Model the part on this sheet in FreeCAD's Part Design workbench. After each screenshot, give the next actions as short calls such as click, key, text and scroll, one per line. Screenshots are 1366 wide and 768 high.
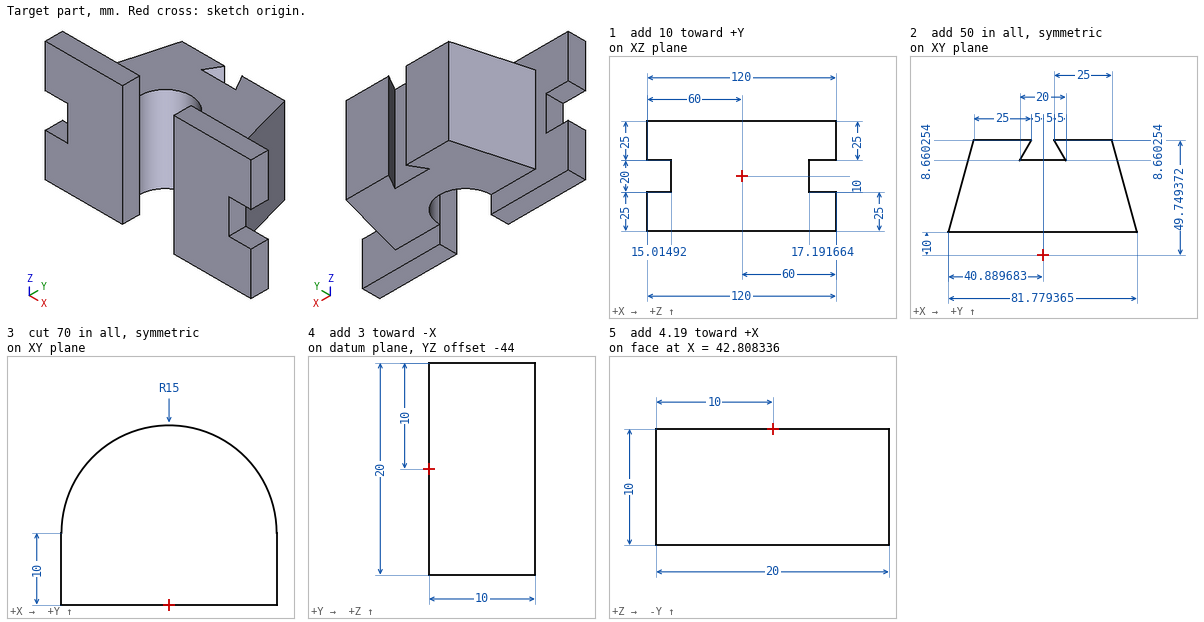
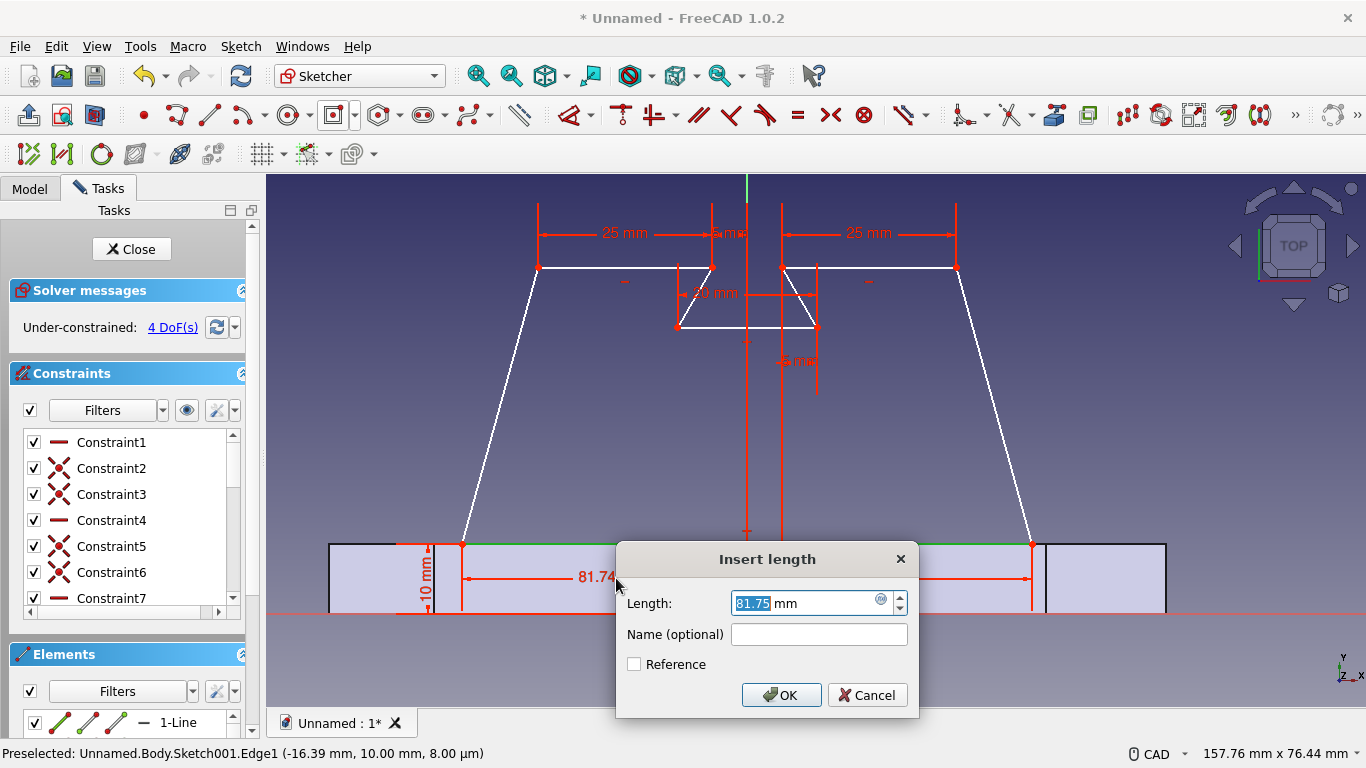
text(81.779365)
key(Return)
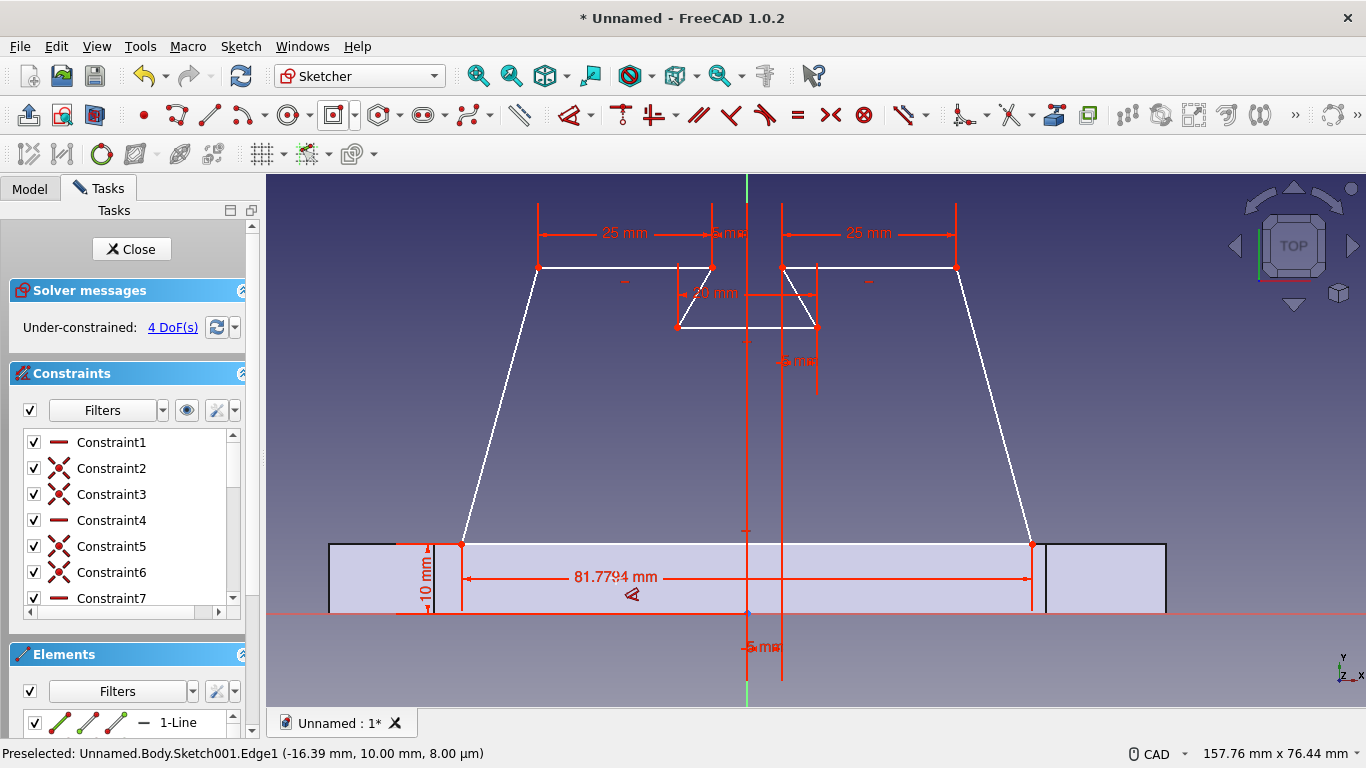
click(793, 286)
click(851, 298)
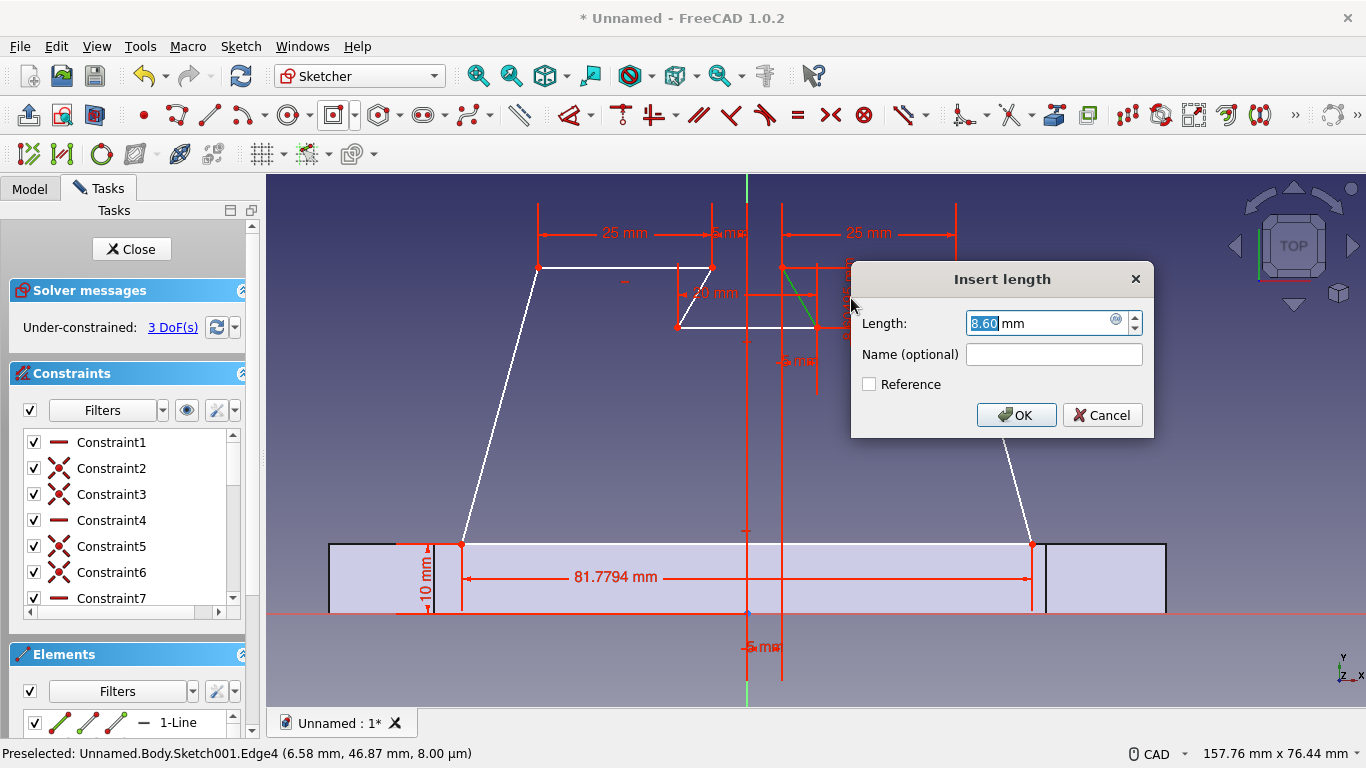
text(8.660254)
key(Return)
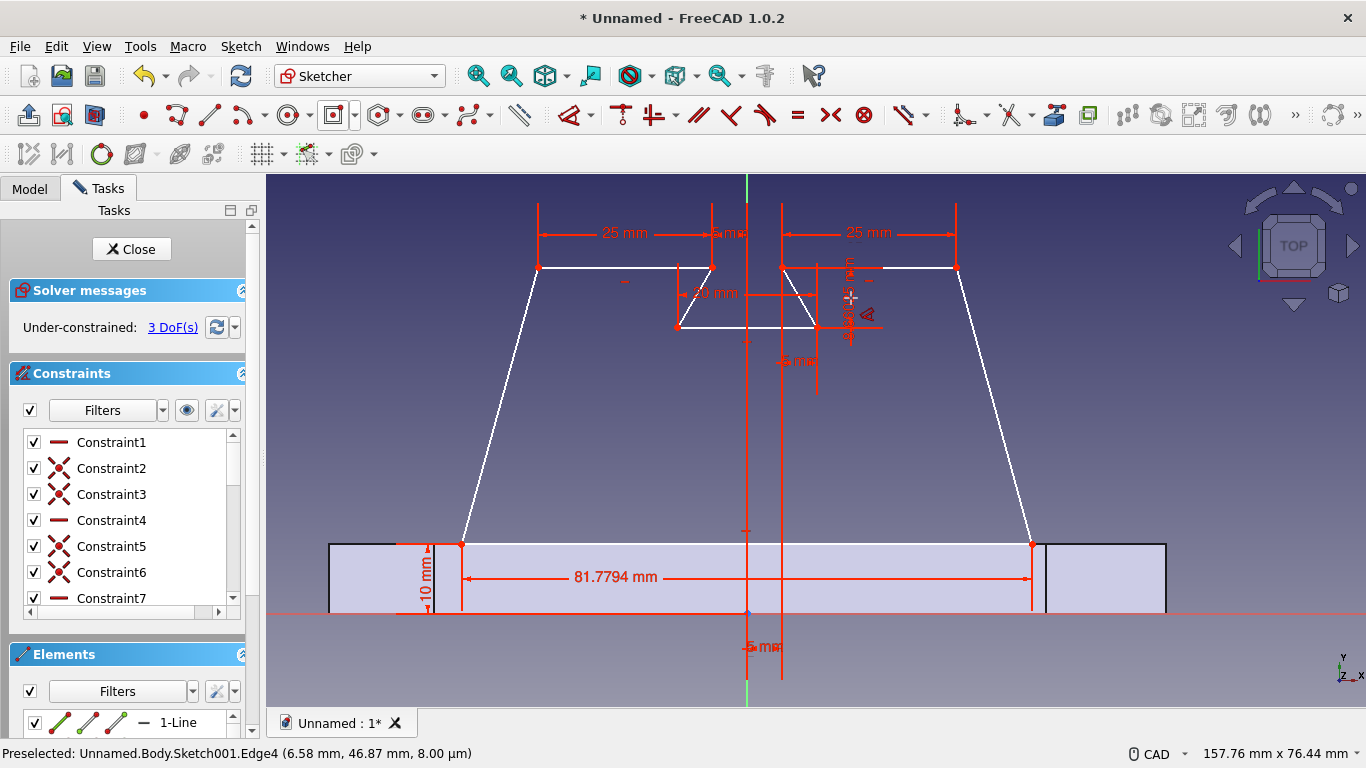
click(688, 310)
click(644, 298)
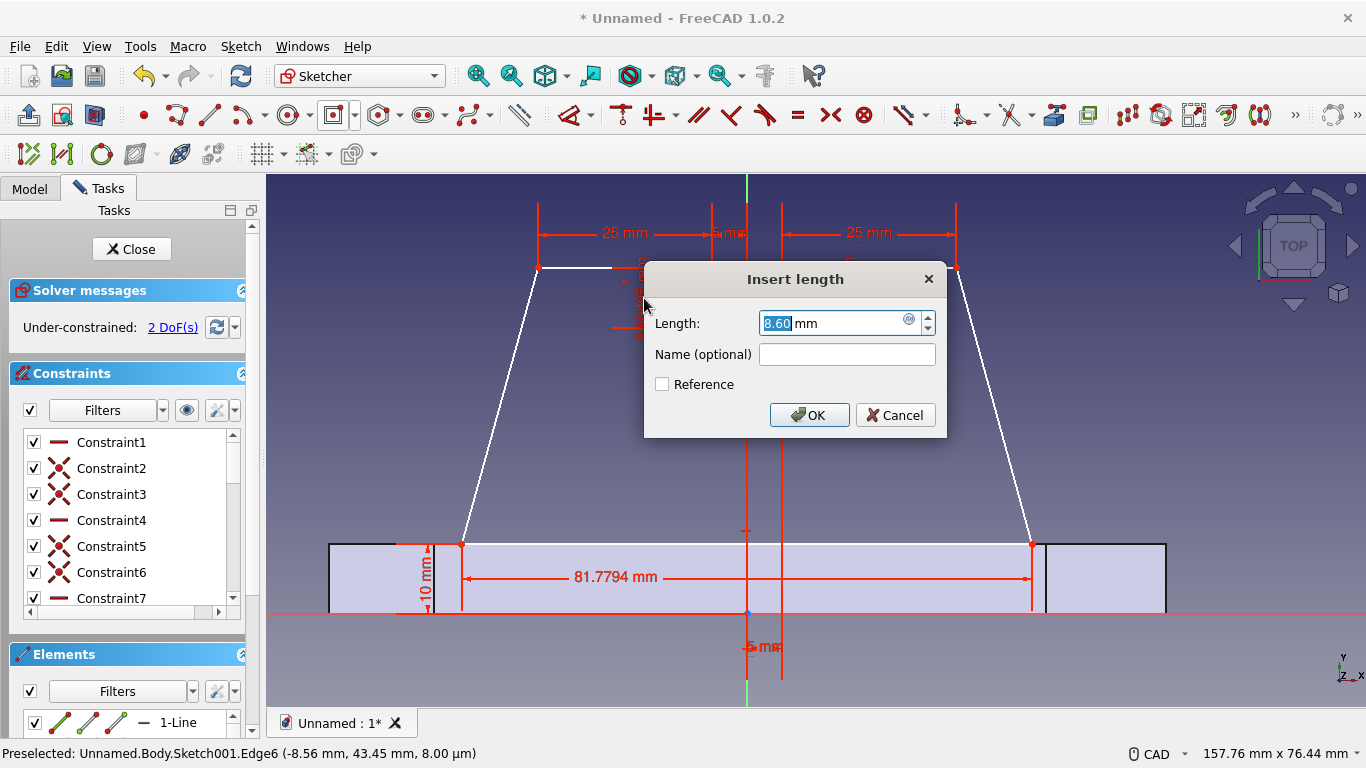
text(8.660254)
key(Return)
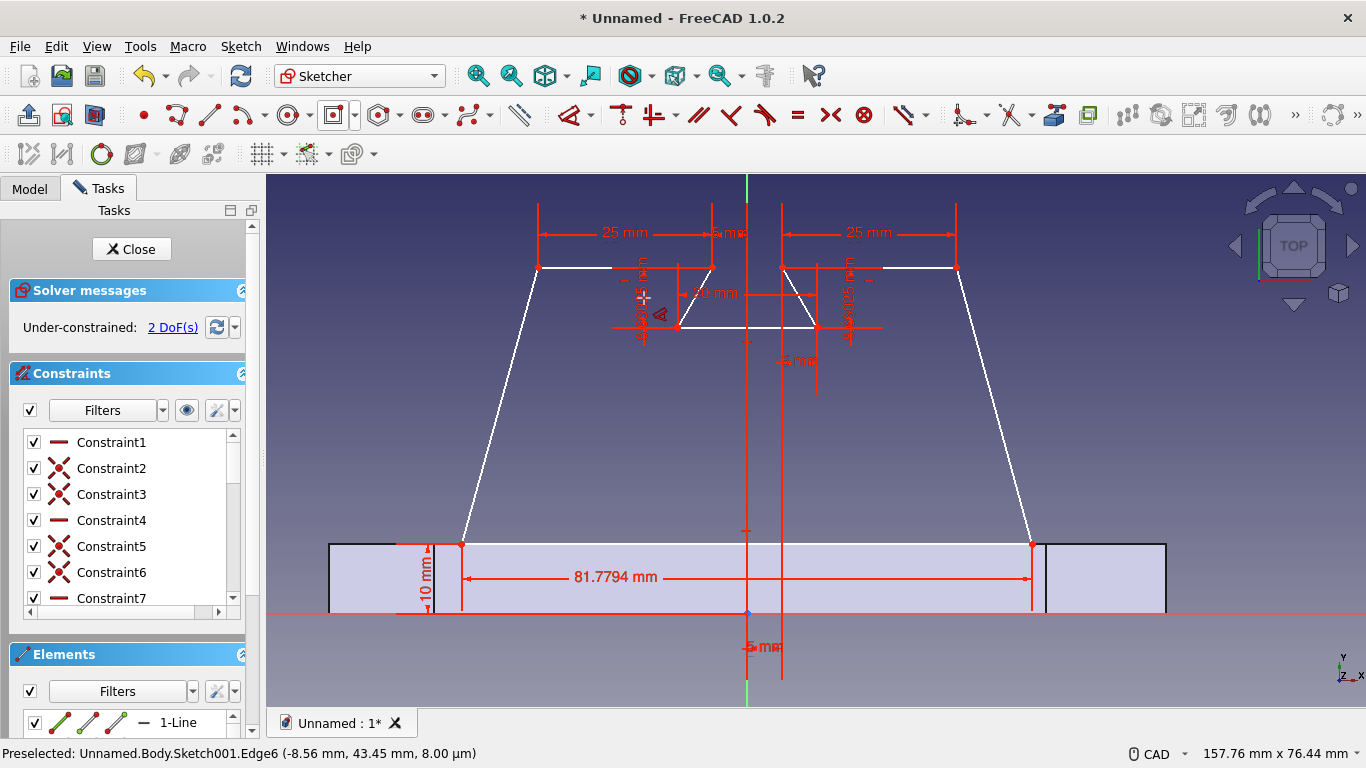
click(462, 544)
click(605, 648)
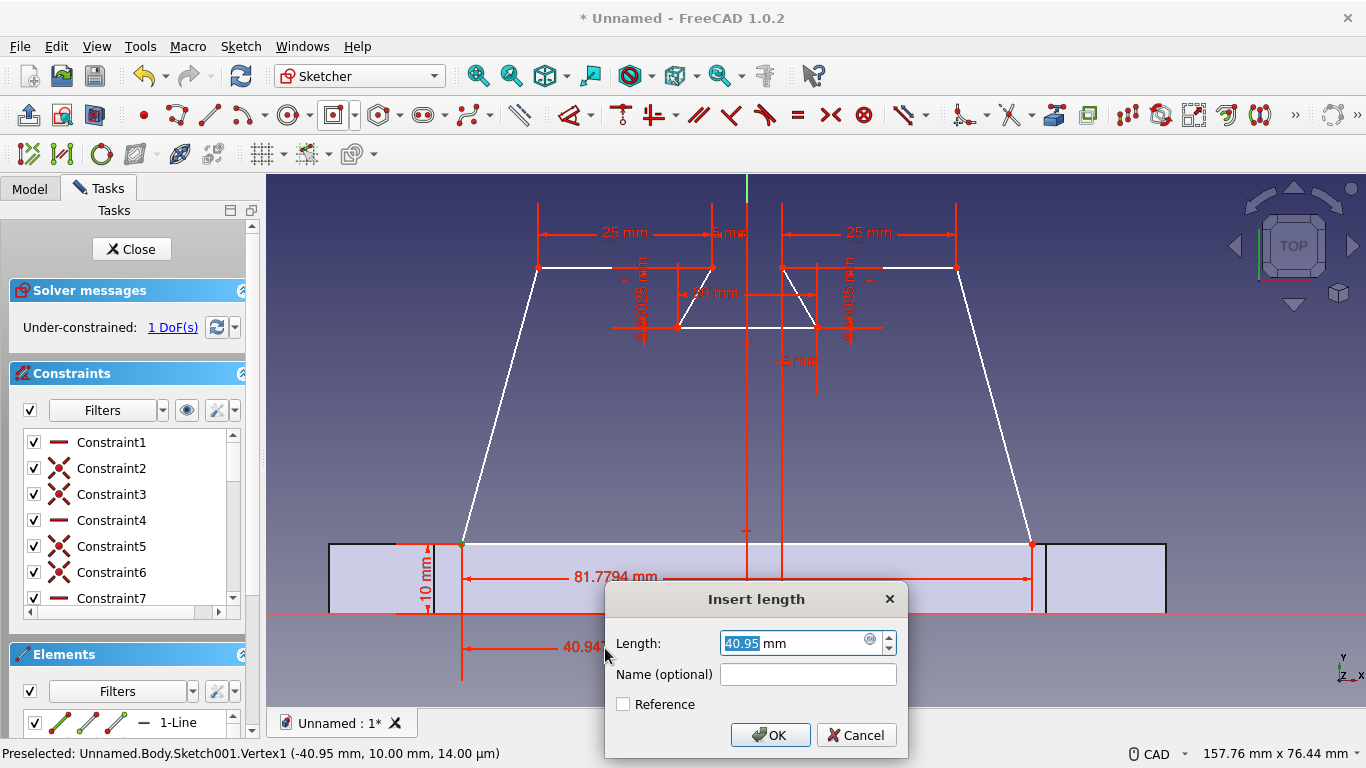
text(40.889683)
key(Return)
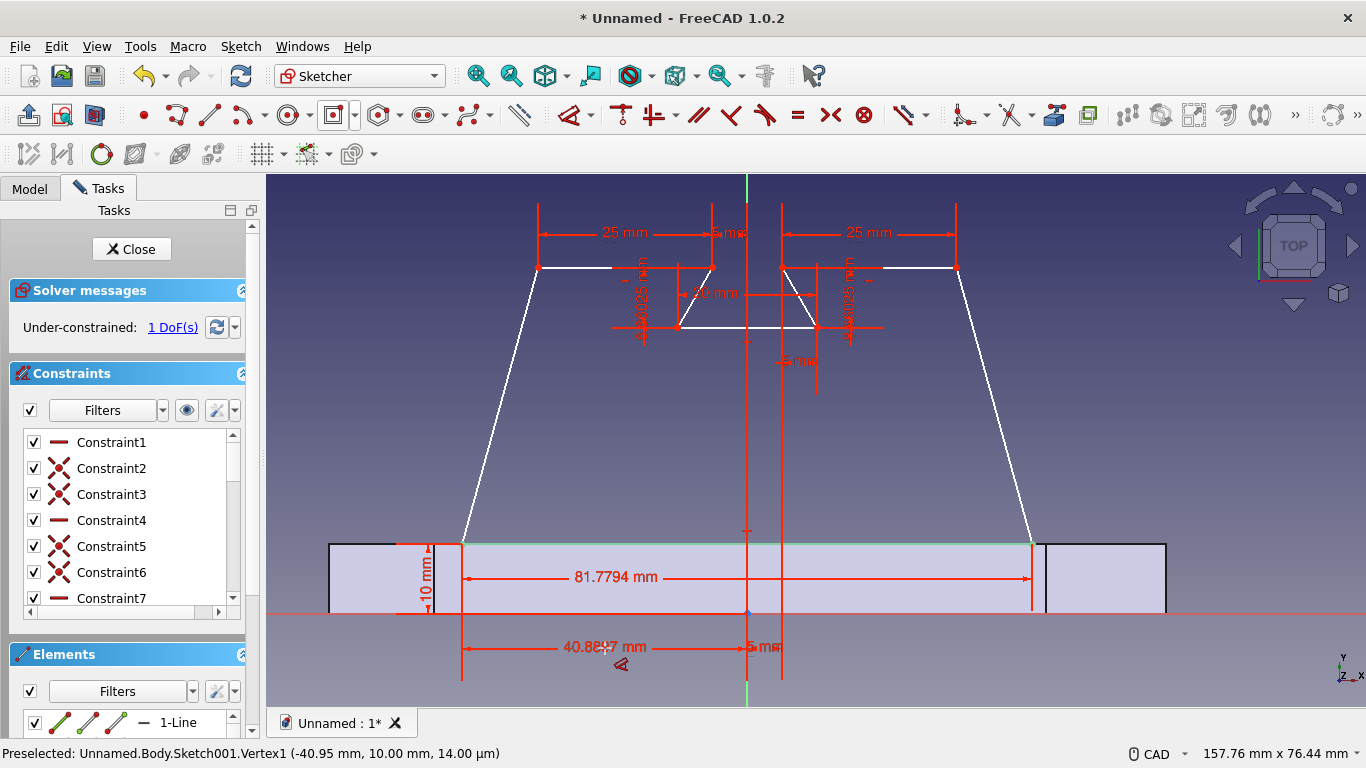
click(956, 268)
click(990, 441)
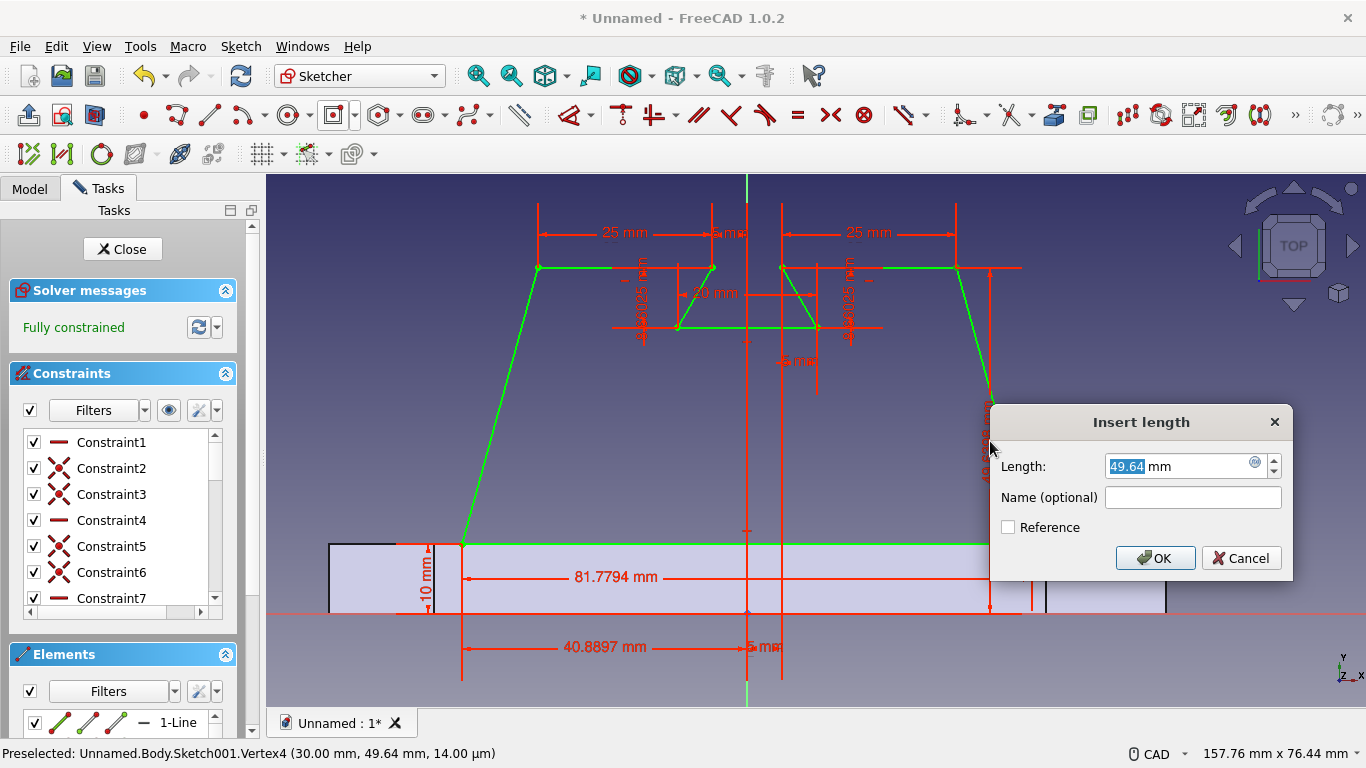
text(49.749372)
key(Return)
key(Escape)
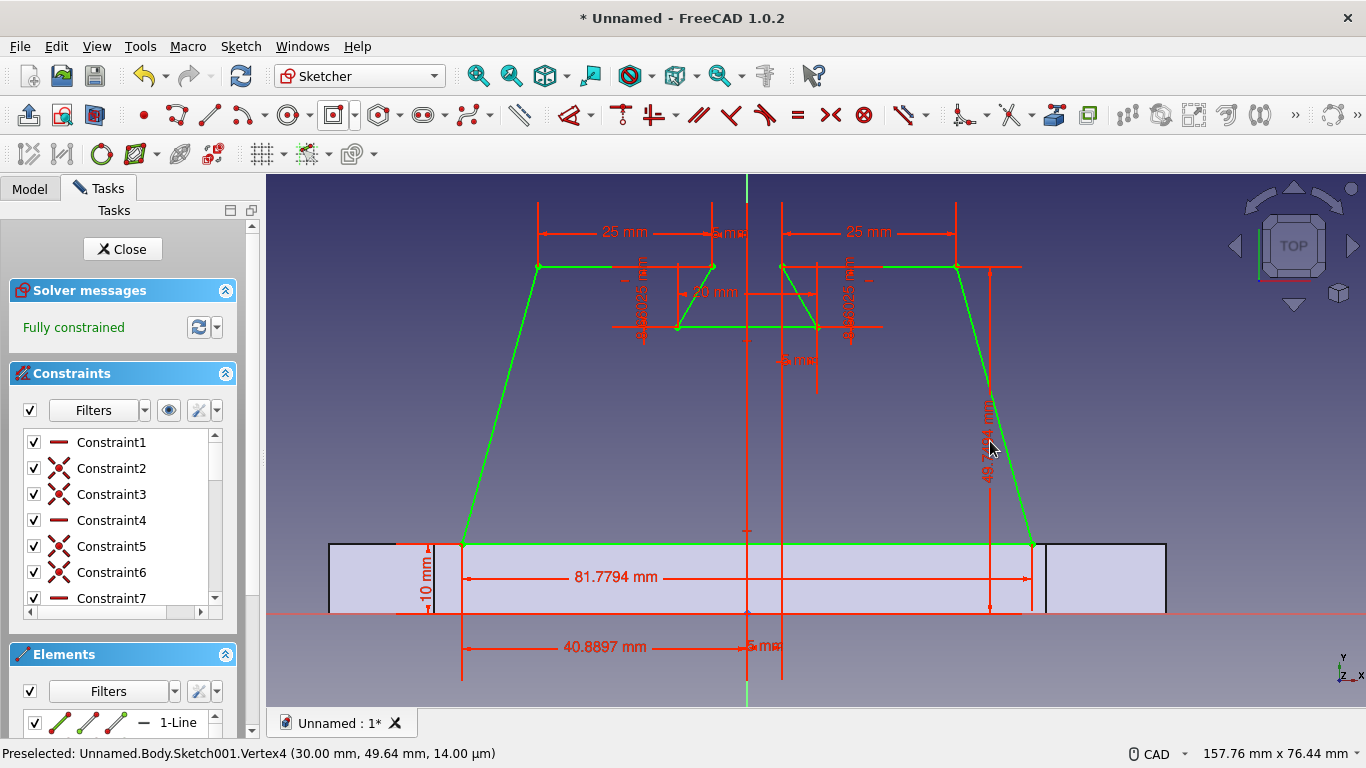
click(123, 249)